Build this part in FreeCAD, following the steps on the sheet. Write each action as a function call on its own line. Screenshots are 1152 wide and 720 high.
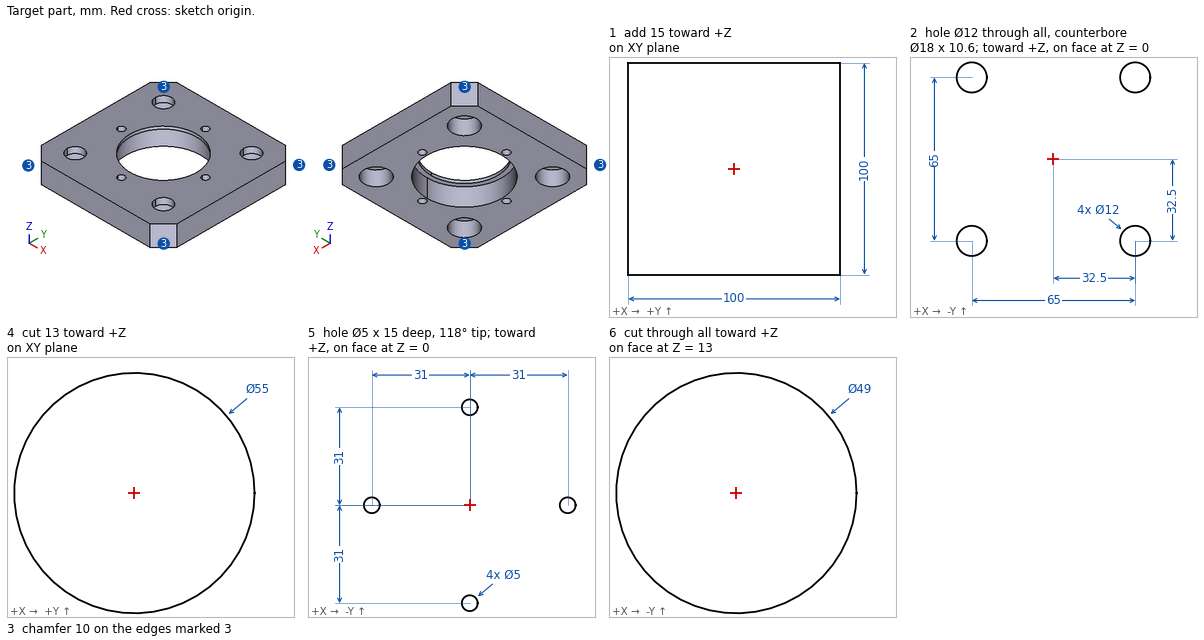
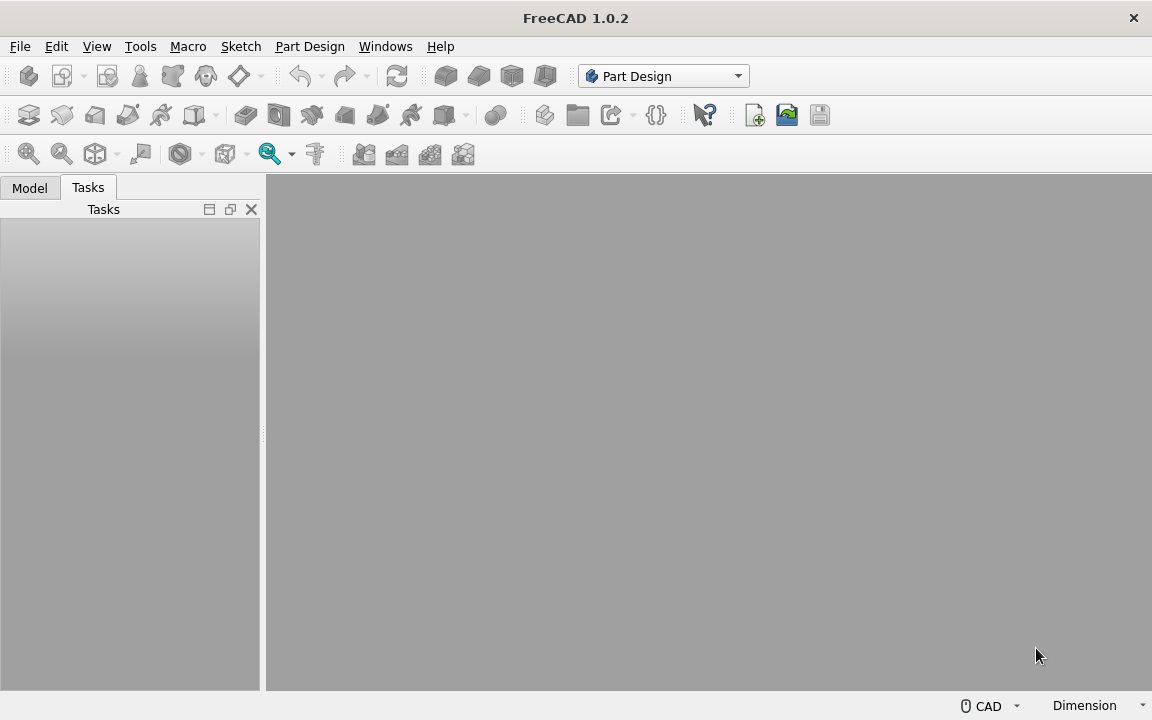
click(754, 116)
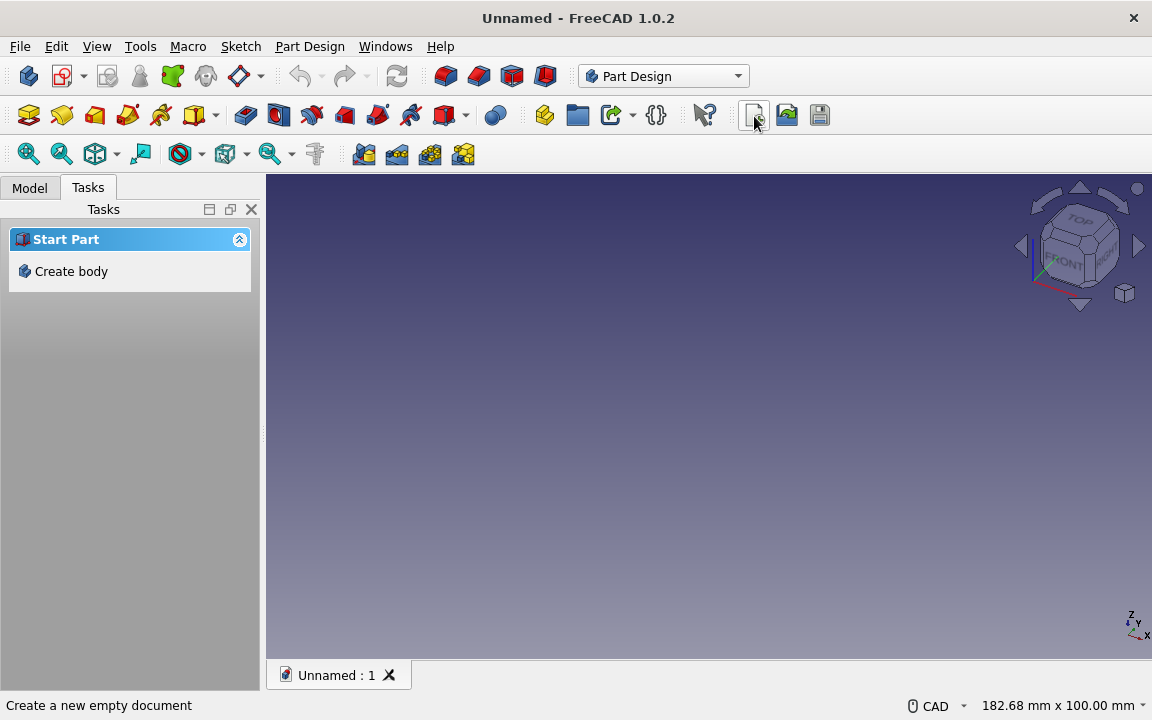
click(62, 76)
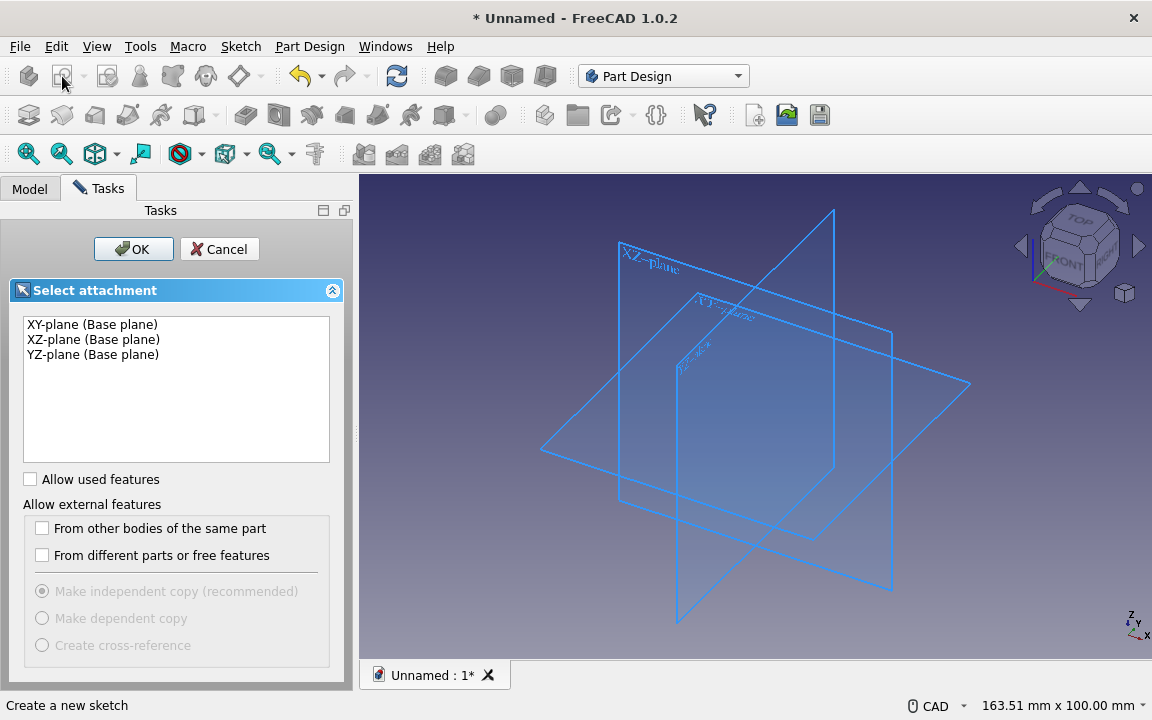
click(84, 324)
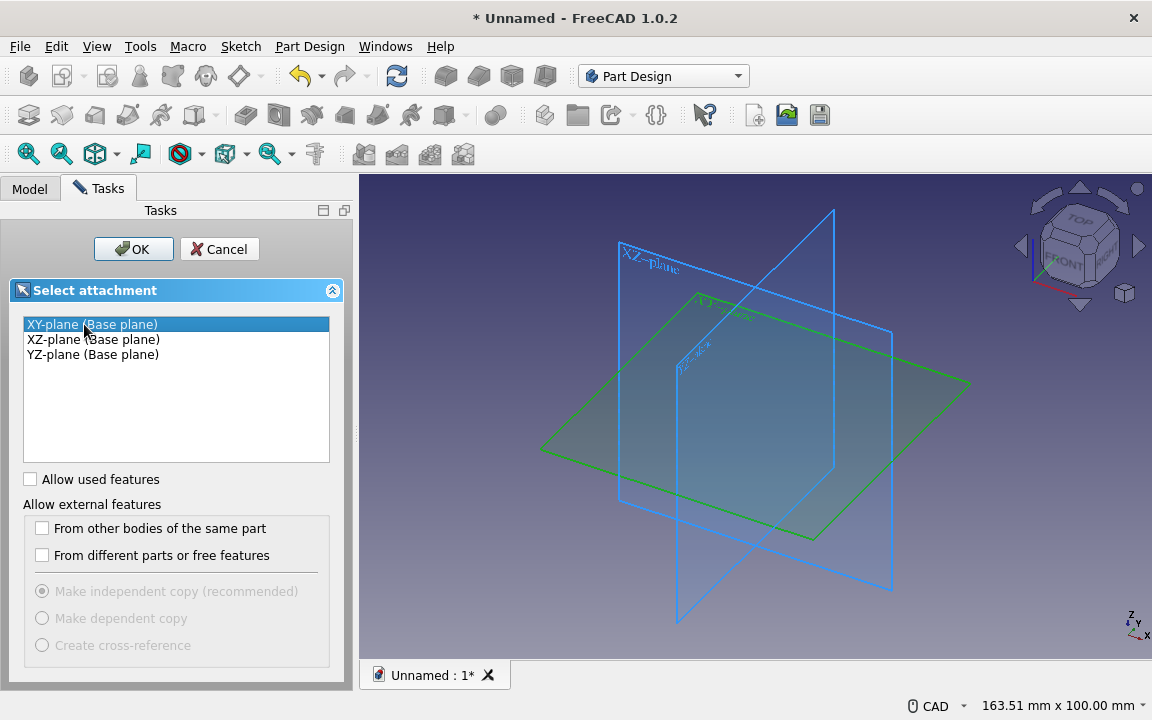
click(134, 249)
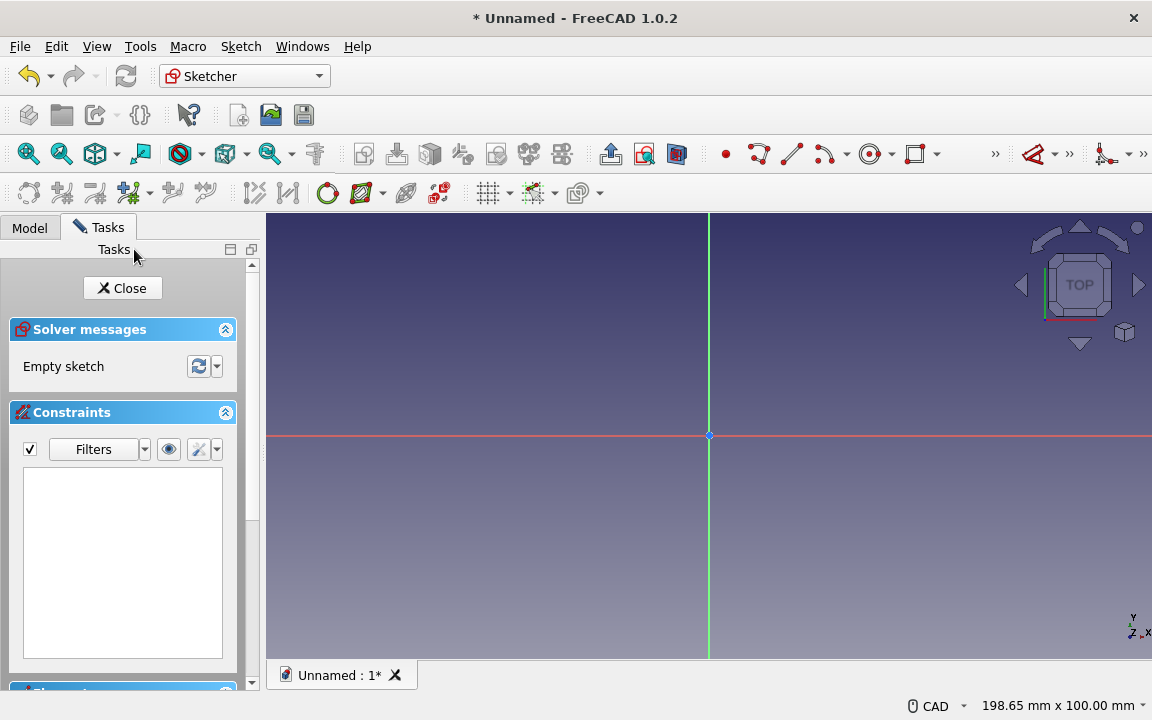
scroll(501, 436, down, 2)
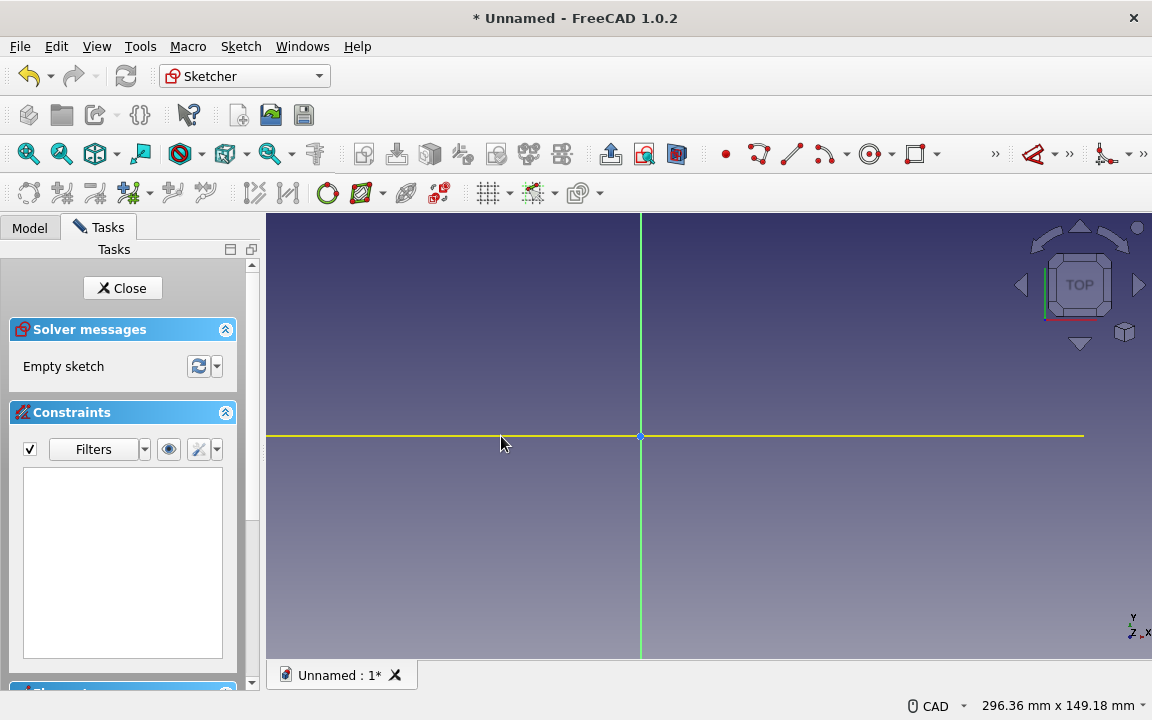
key(g)
key(v)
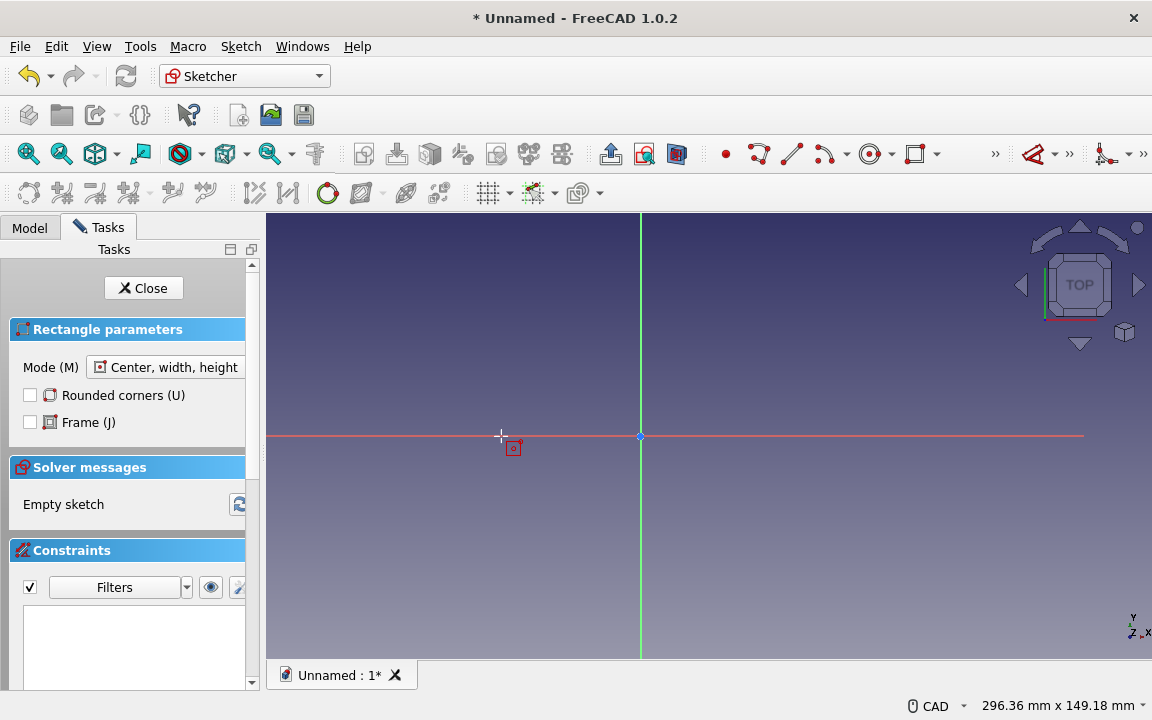
click(641, 436)
move(790, 287)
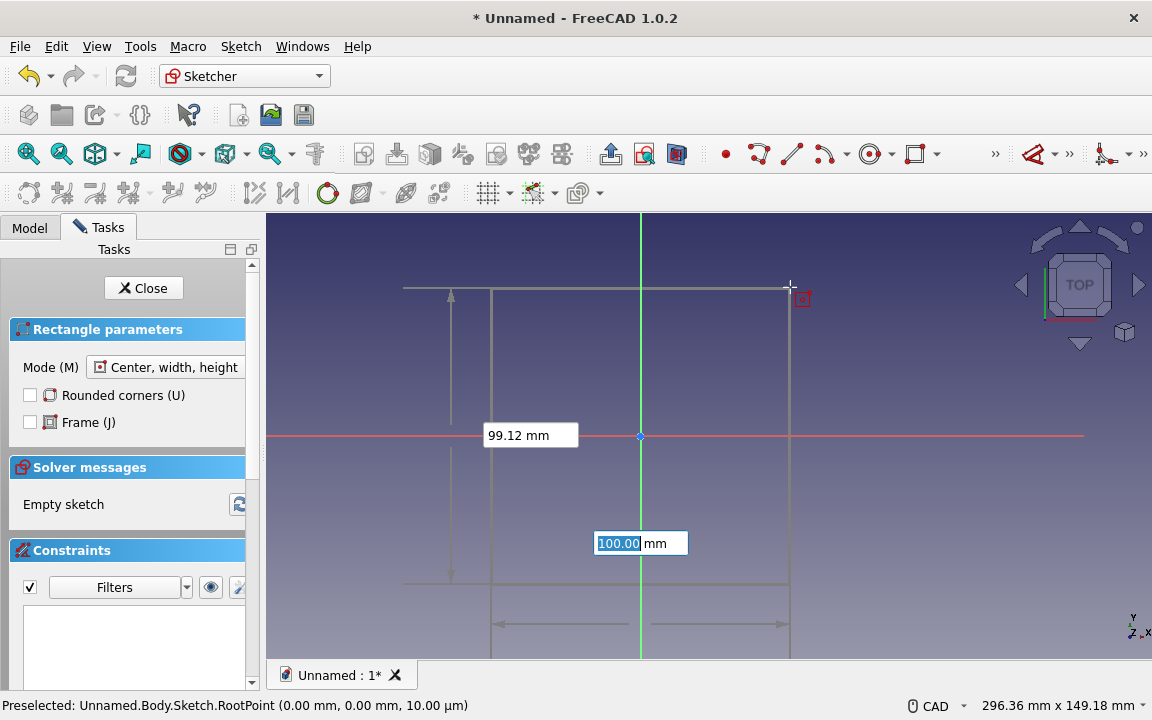
text(100)
key(Tab)
text(100)
key(Return)
key(Escape)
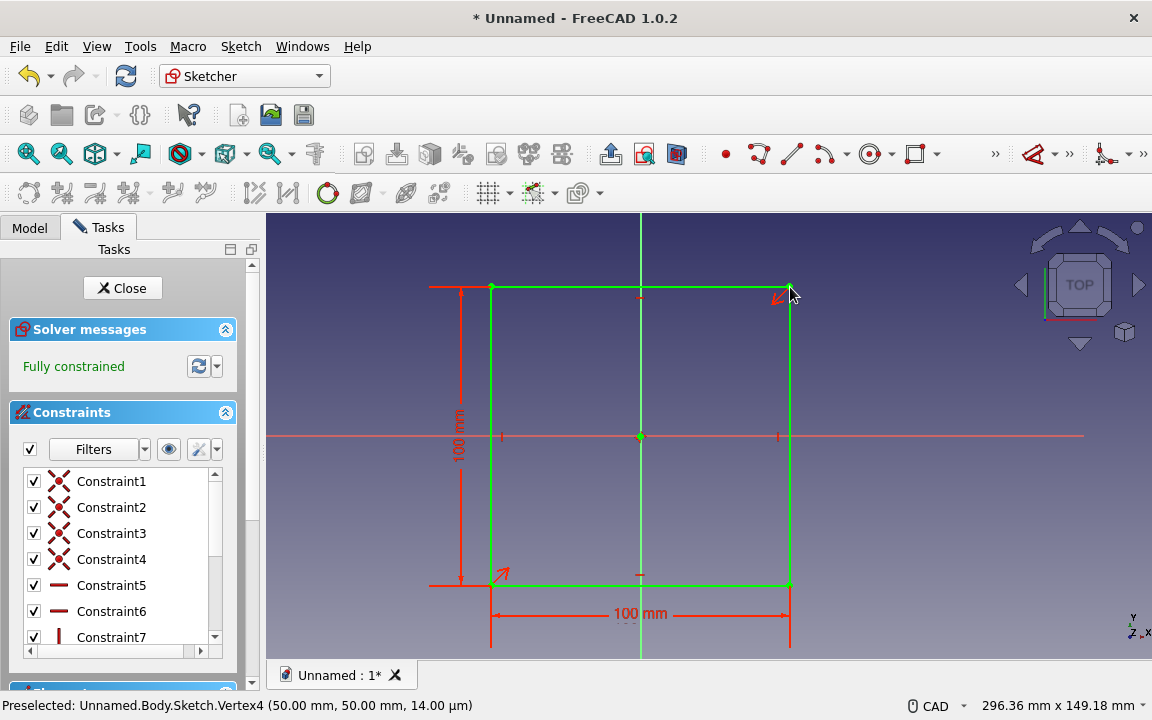
click(123, 288)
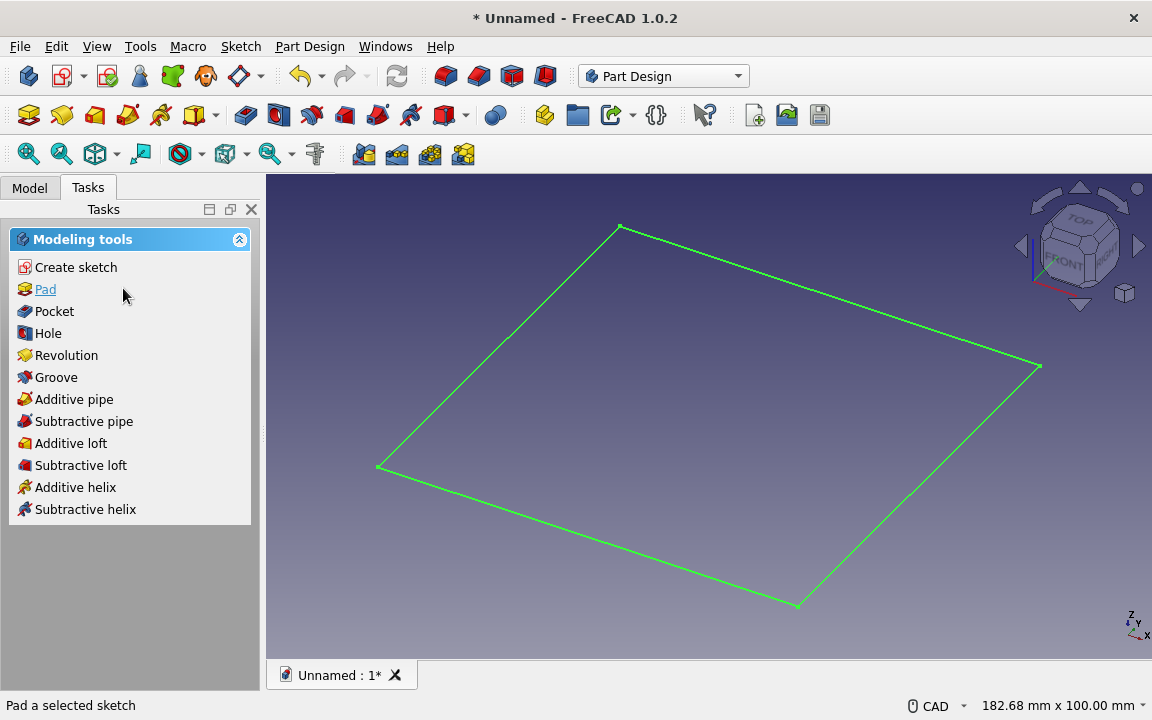
click(29, 116)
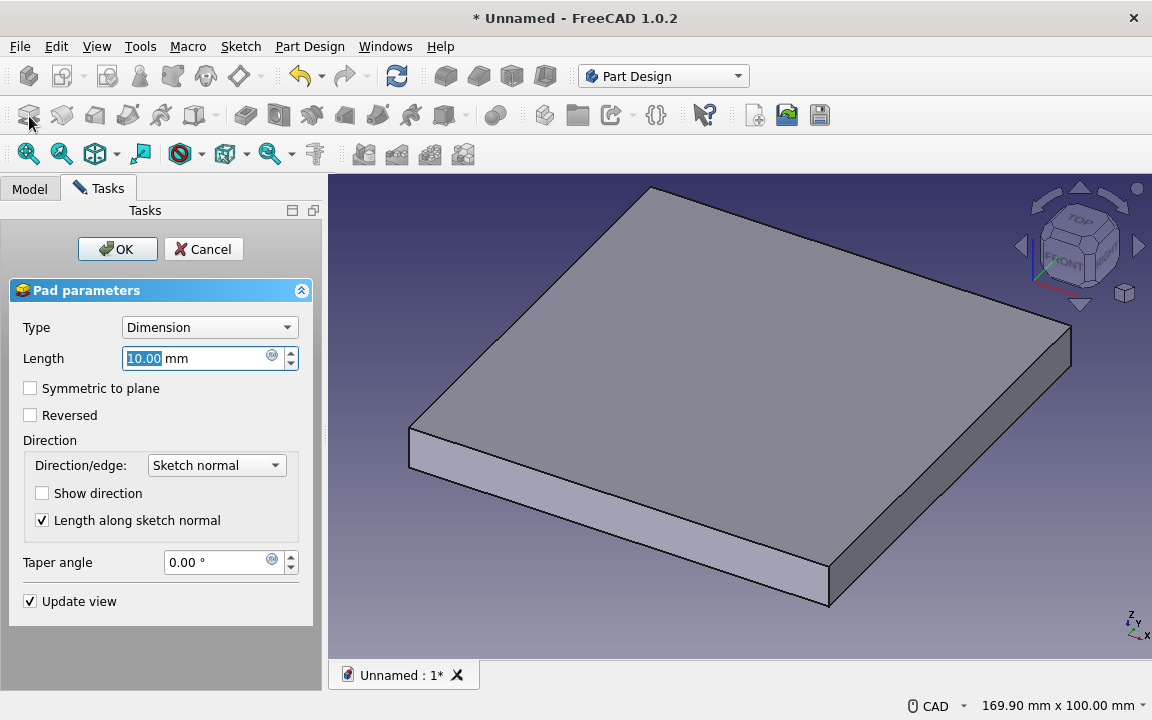
text(15)
key(Tab)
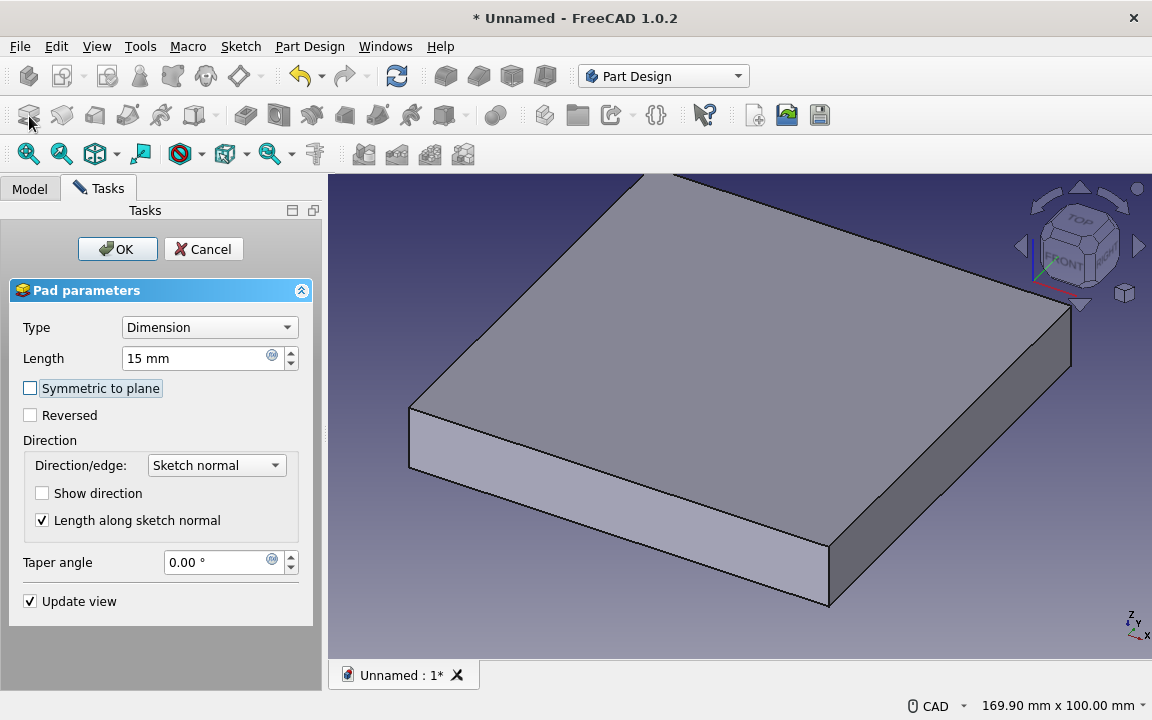
click(118, 249)